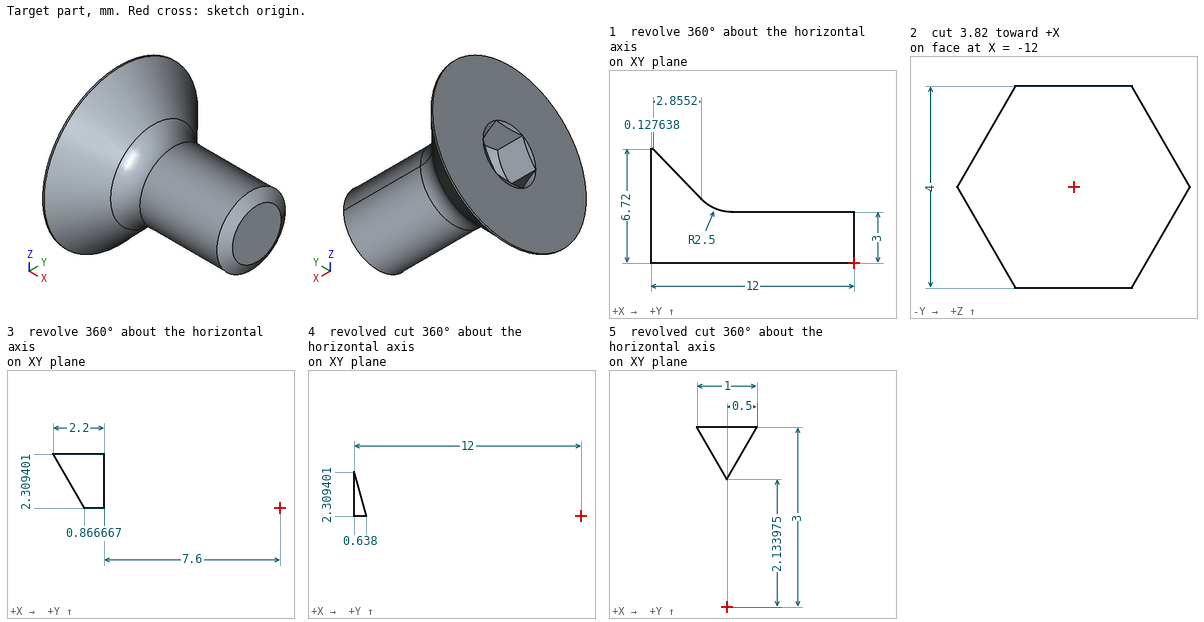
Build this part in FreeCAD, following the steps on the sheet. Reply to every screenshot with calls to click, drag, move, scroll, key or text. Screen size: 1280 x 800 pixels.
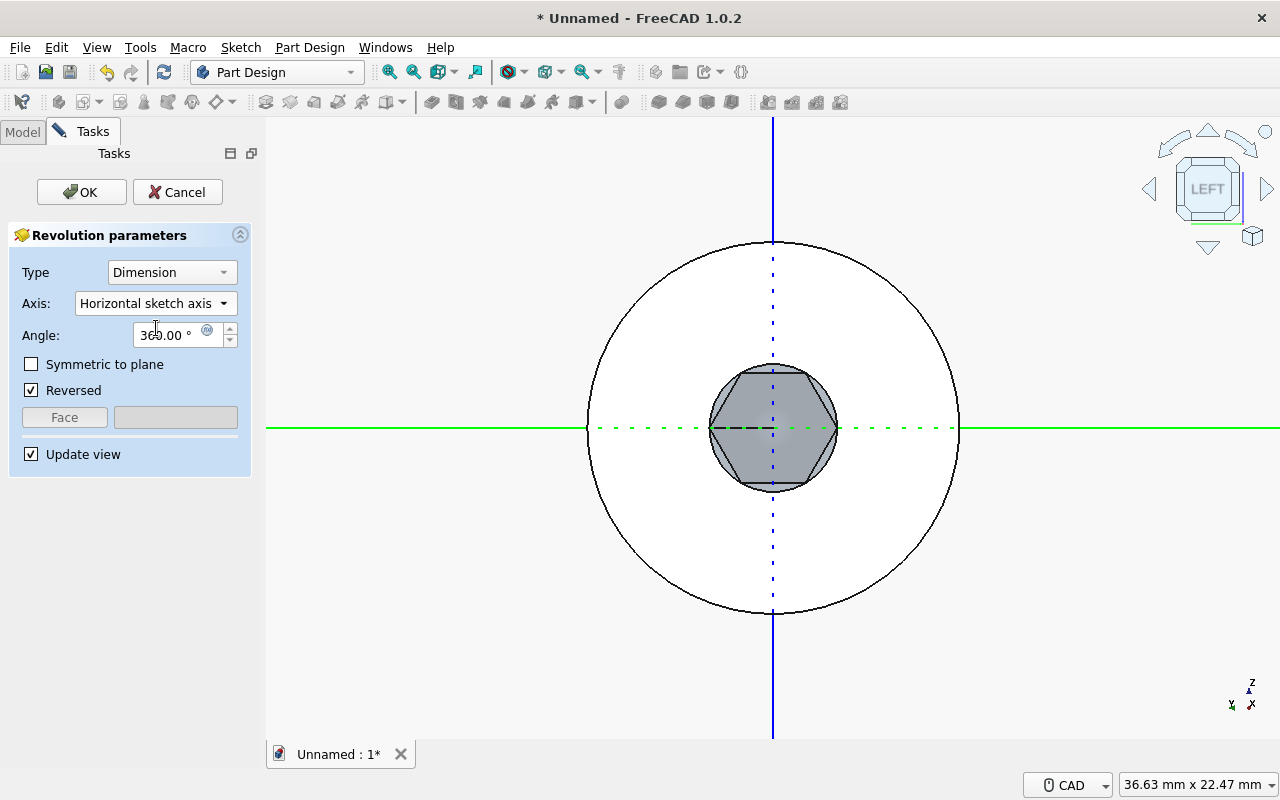
click(82, 192)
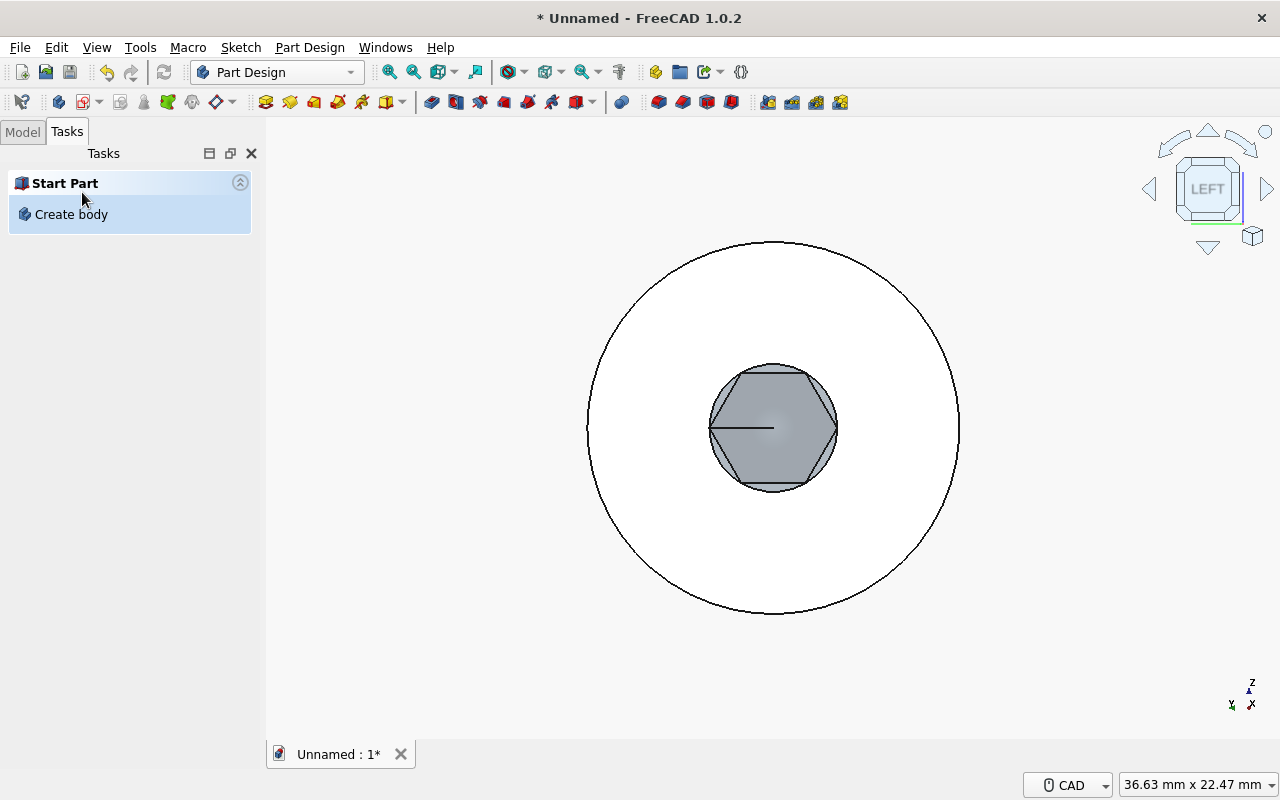
click(84, 102)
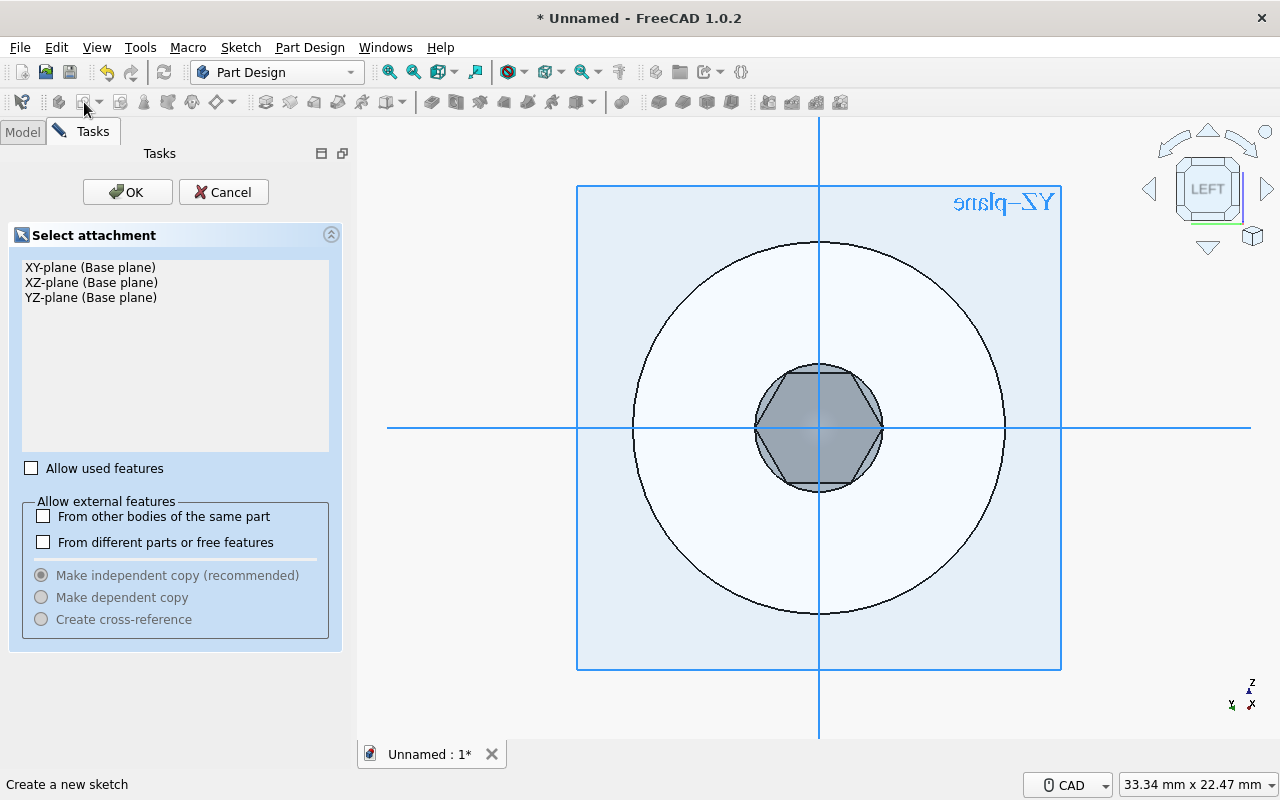
click(82, 268)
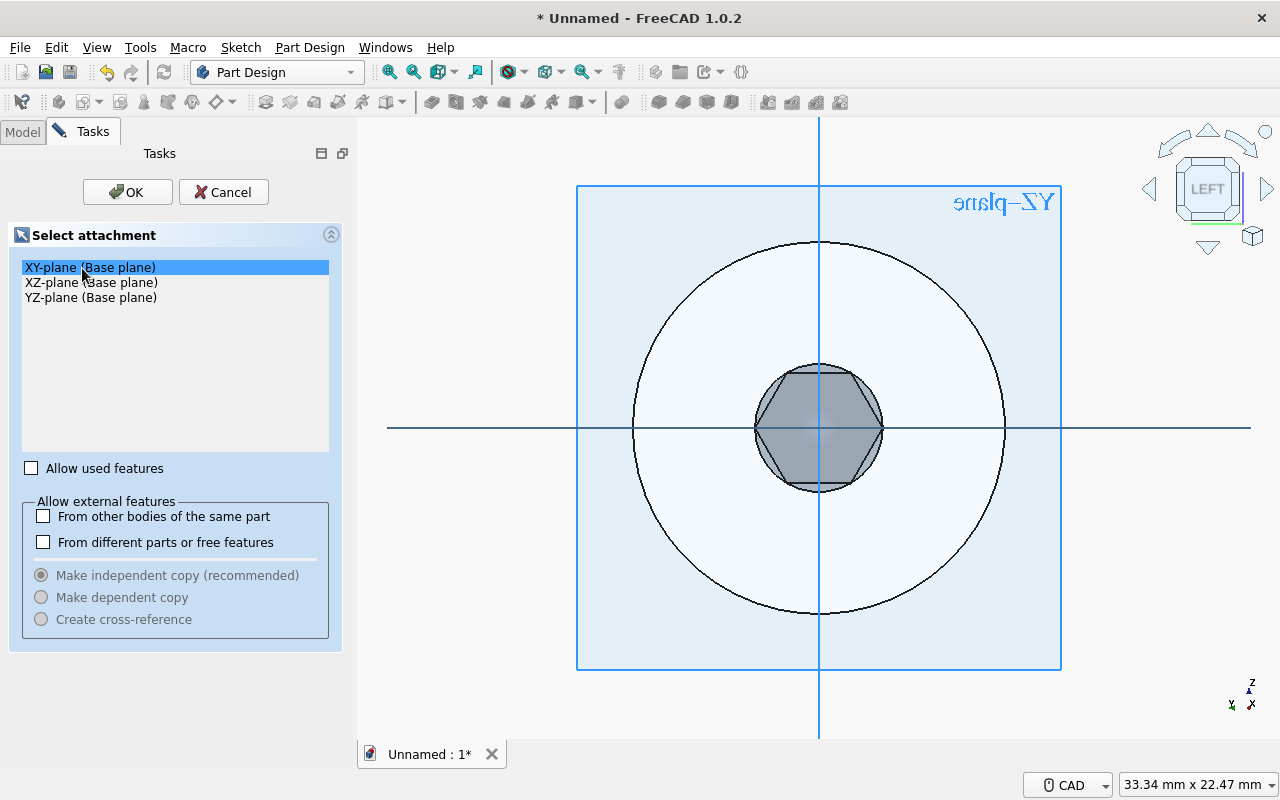
click(128, 192)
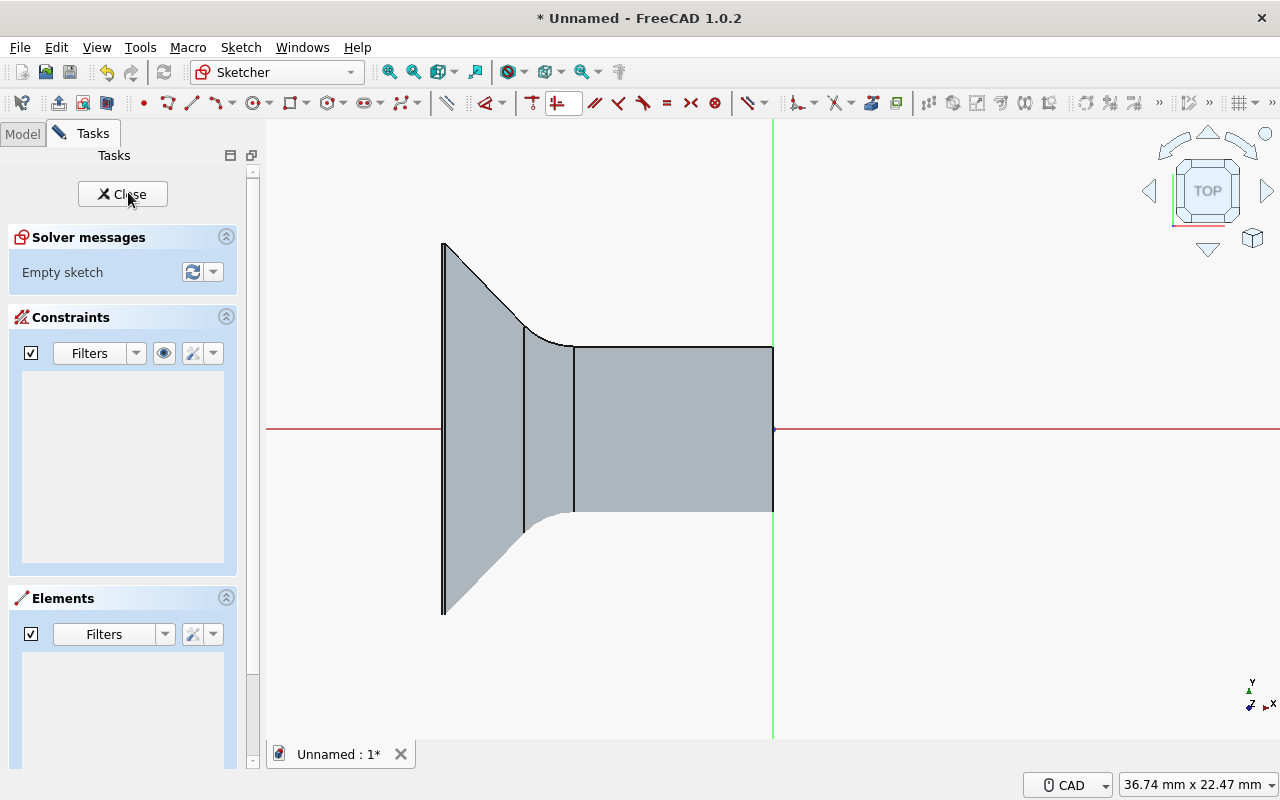
key(q)
key(s)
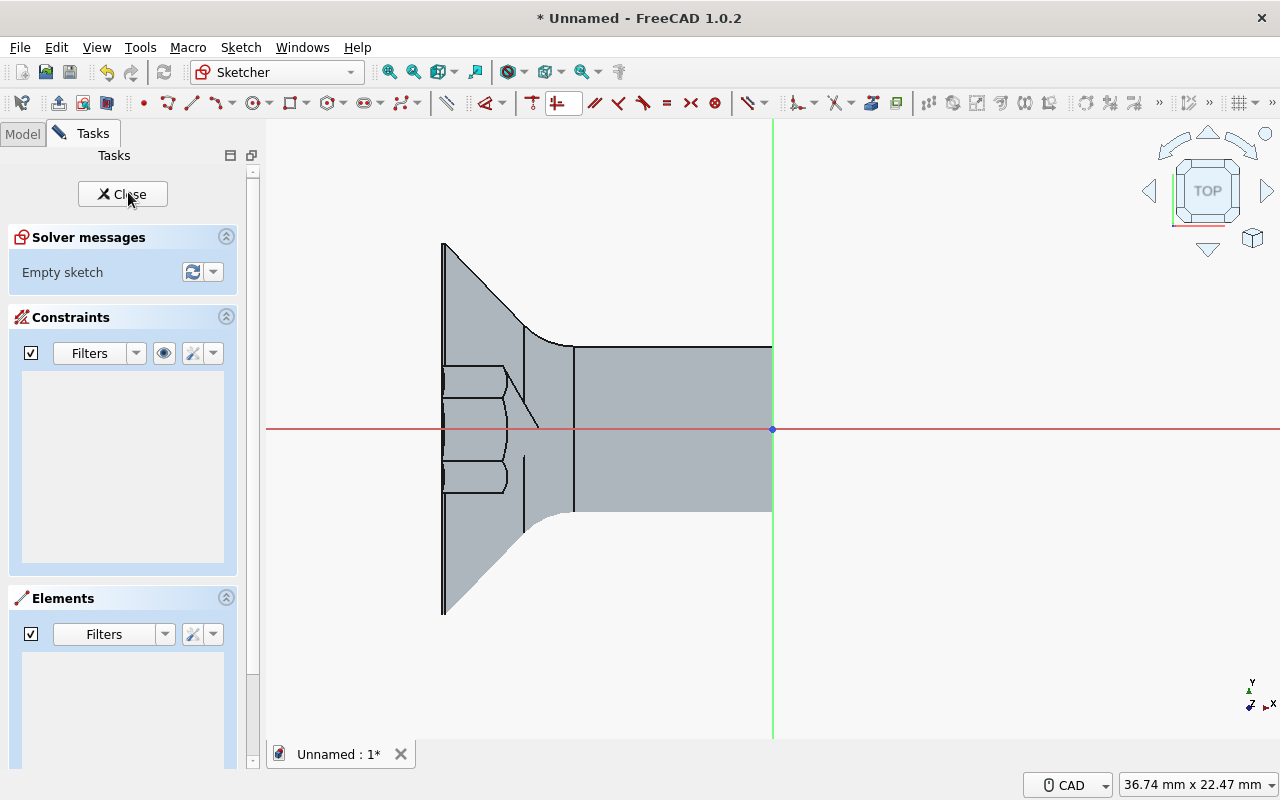
scroll(777, 354, up, 14)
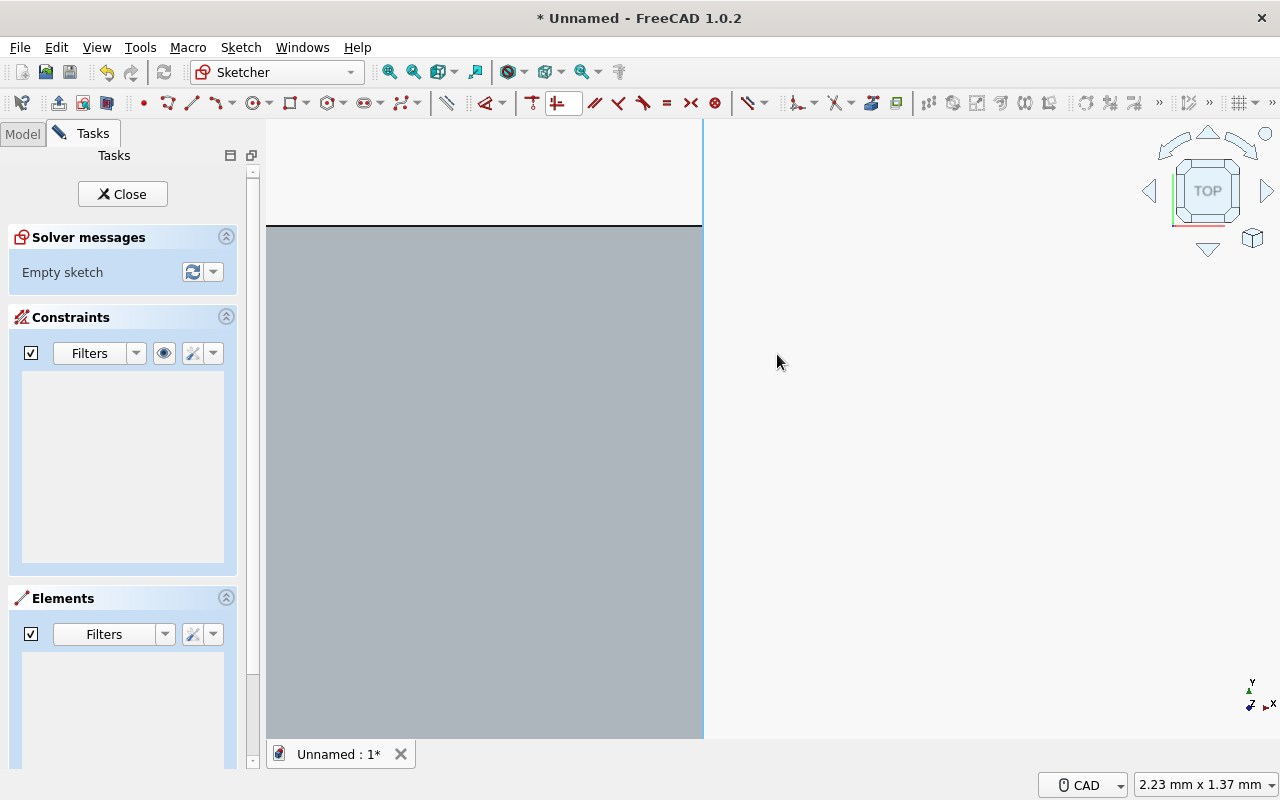
click(168, 104)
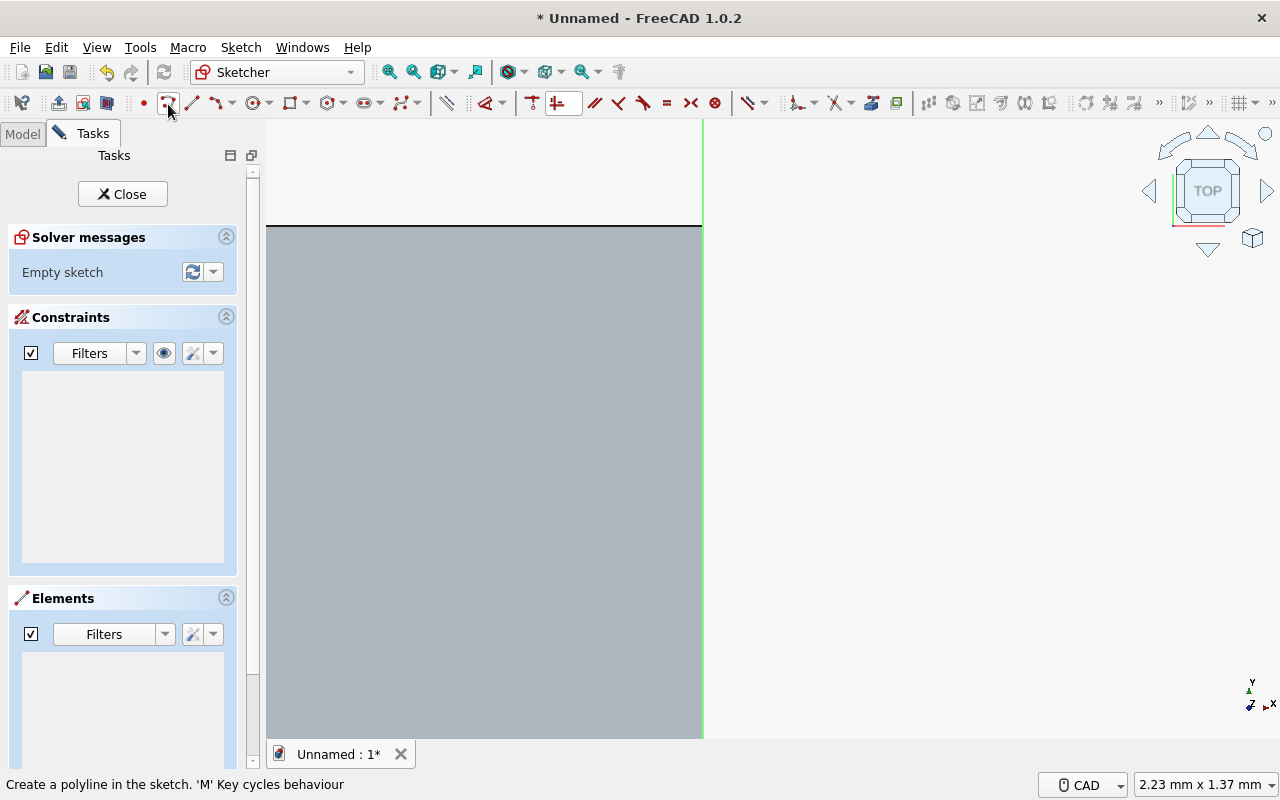
click(703, 619)
click(930, 226)
click(477, 226)
click(703, 620)
key(Escape)
key(Escape)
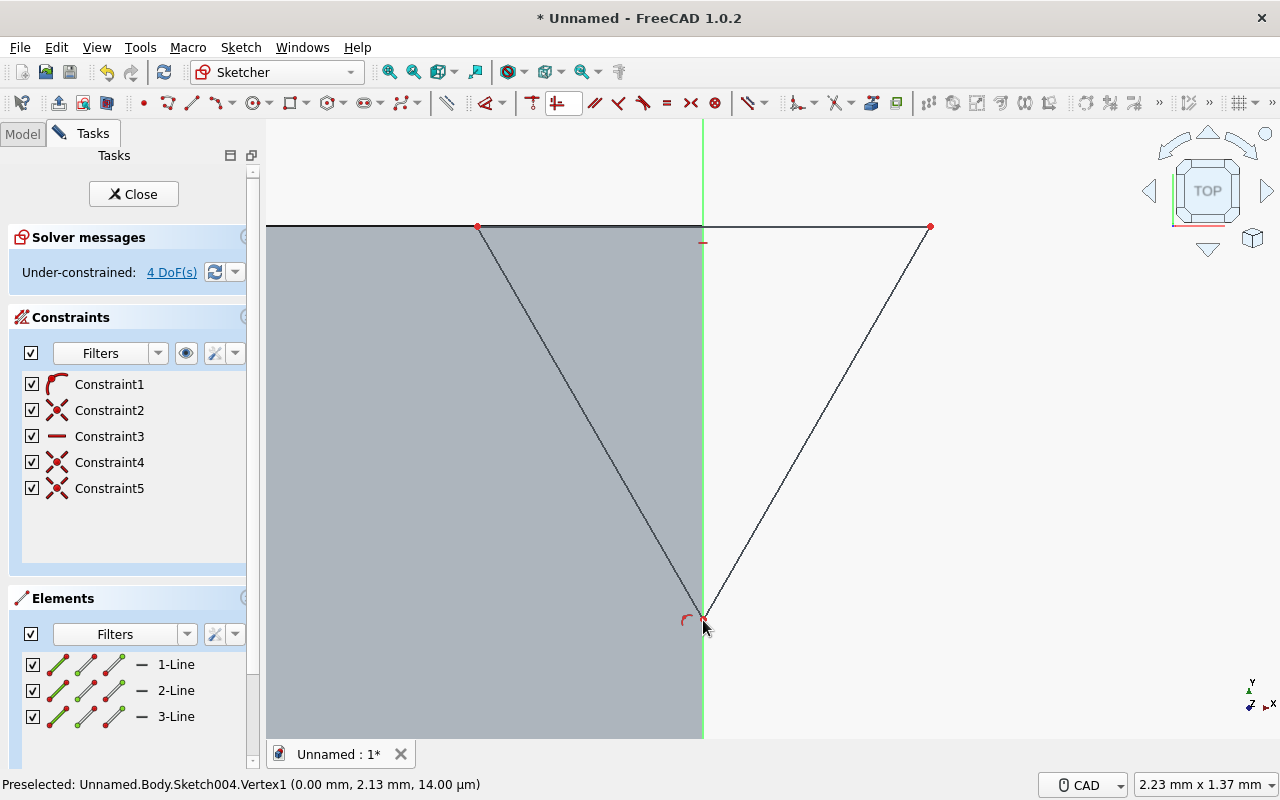
click(486, 104)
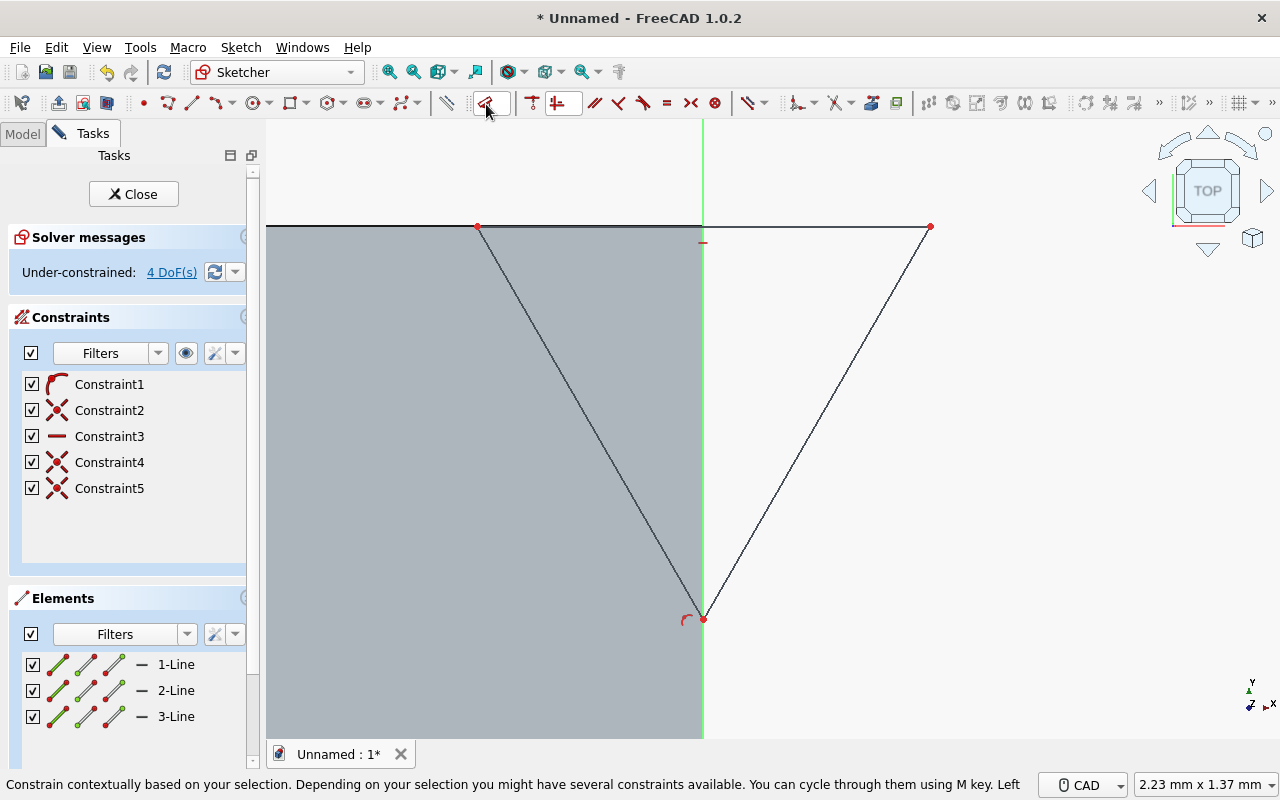
click(794, 227)
click(599, 193)